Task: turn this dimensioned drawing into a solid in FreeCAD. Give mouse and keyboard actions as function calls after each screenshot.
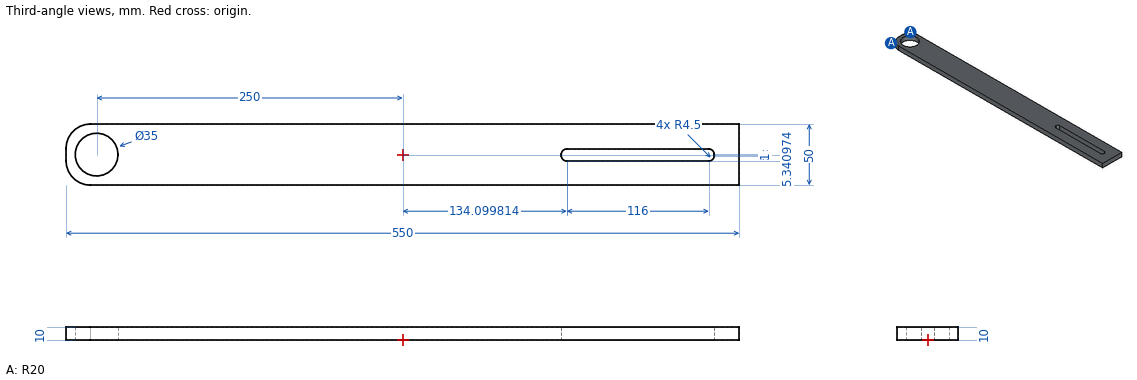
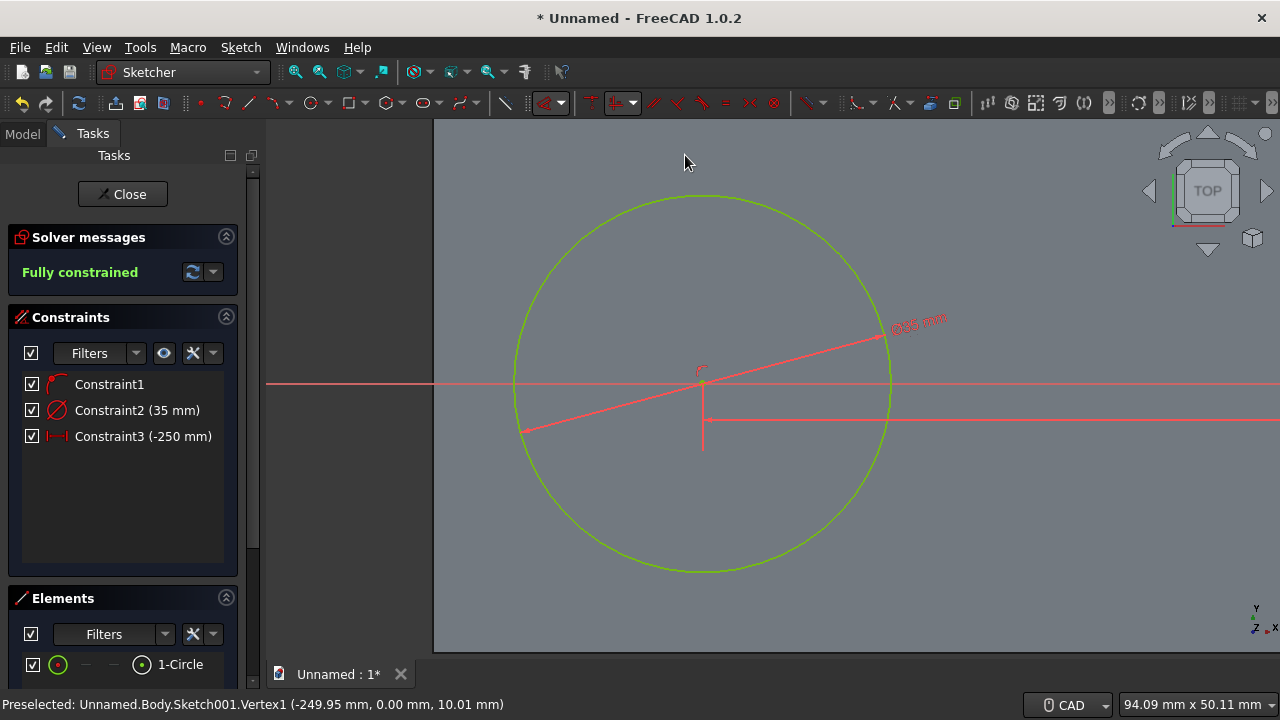
click(123, 194)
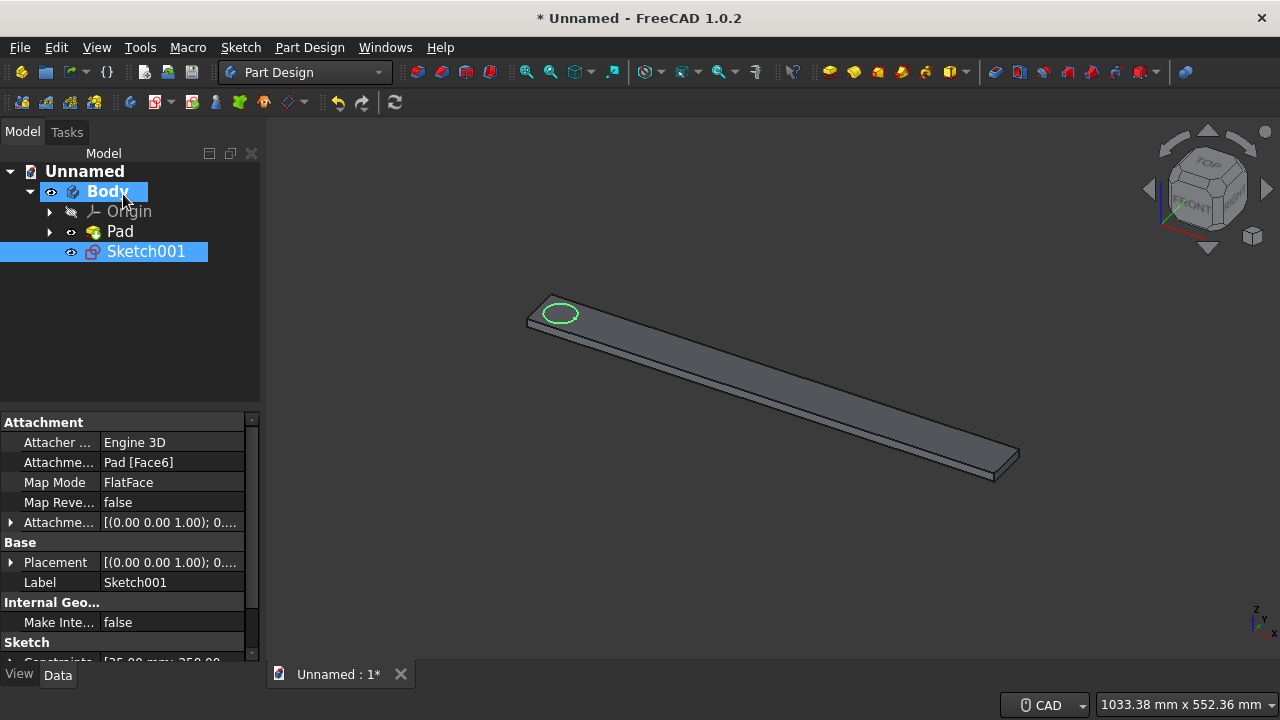
click(996, 72)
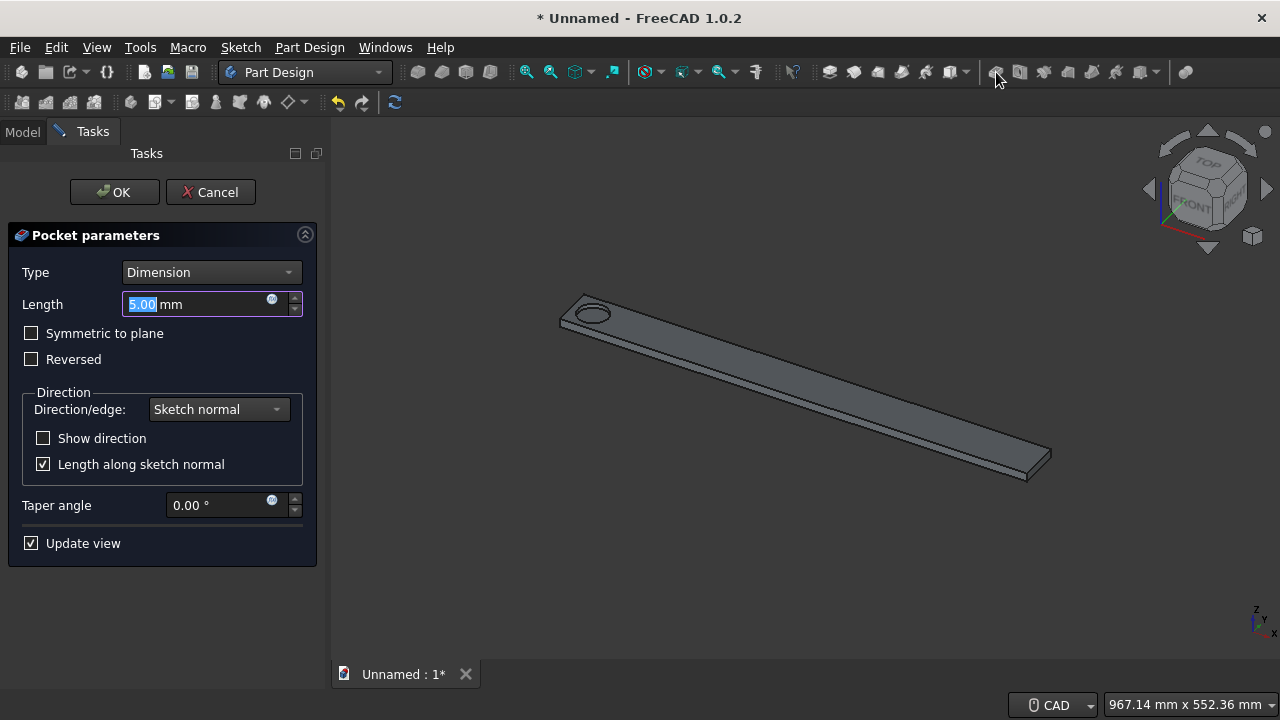
text(10)
key(Tab)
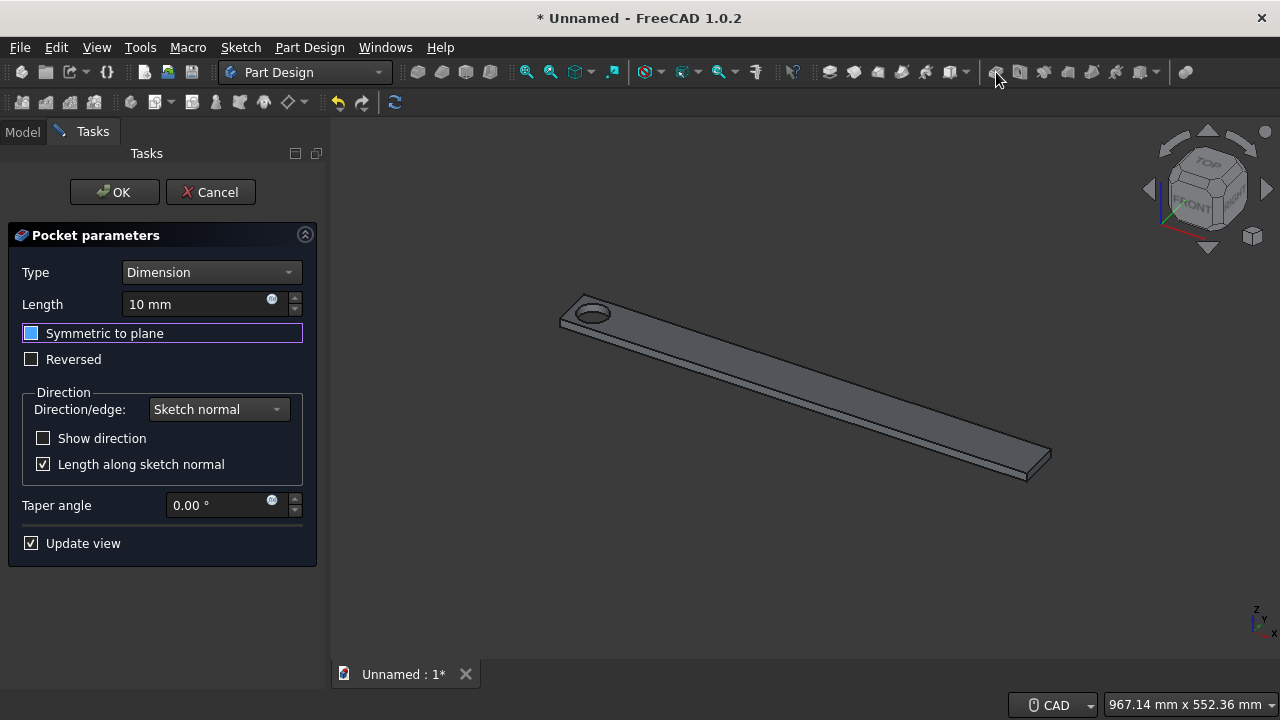
click(115, 192)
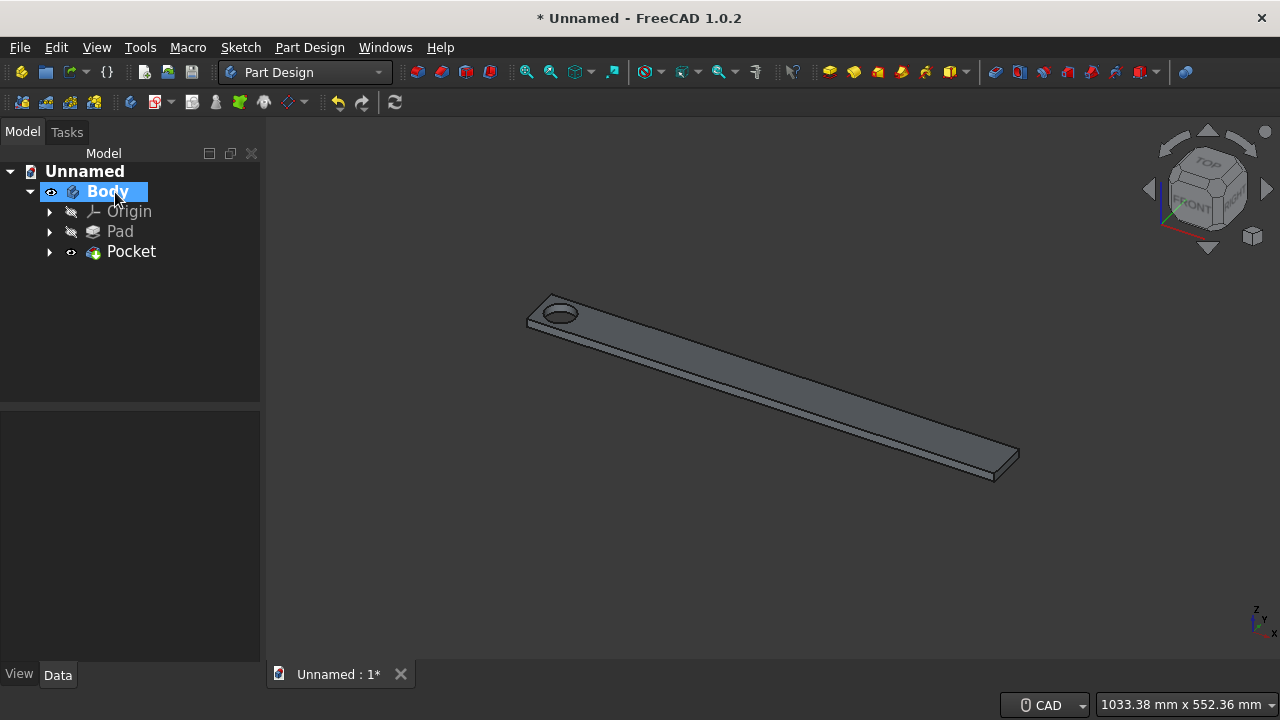
click(973, 449)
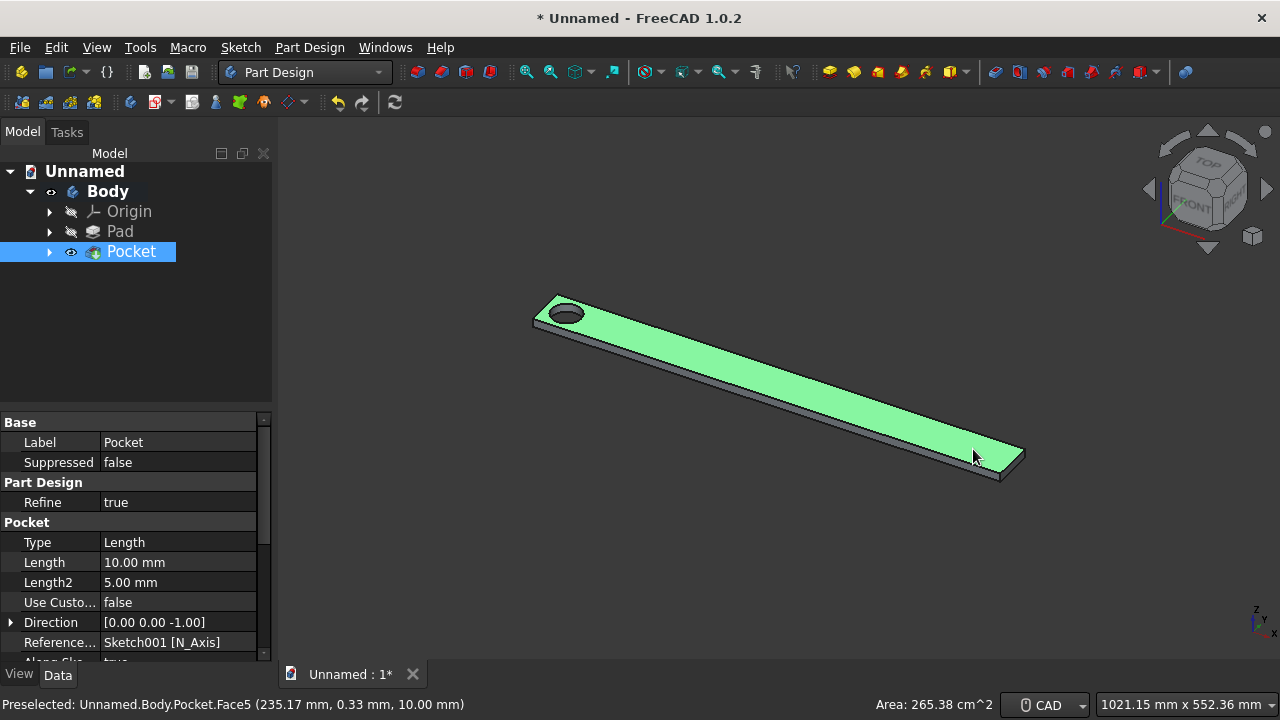
click(156, 102)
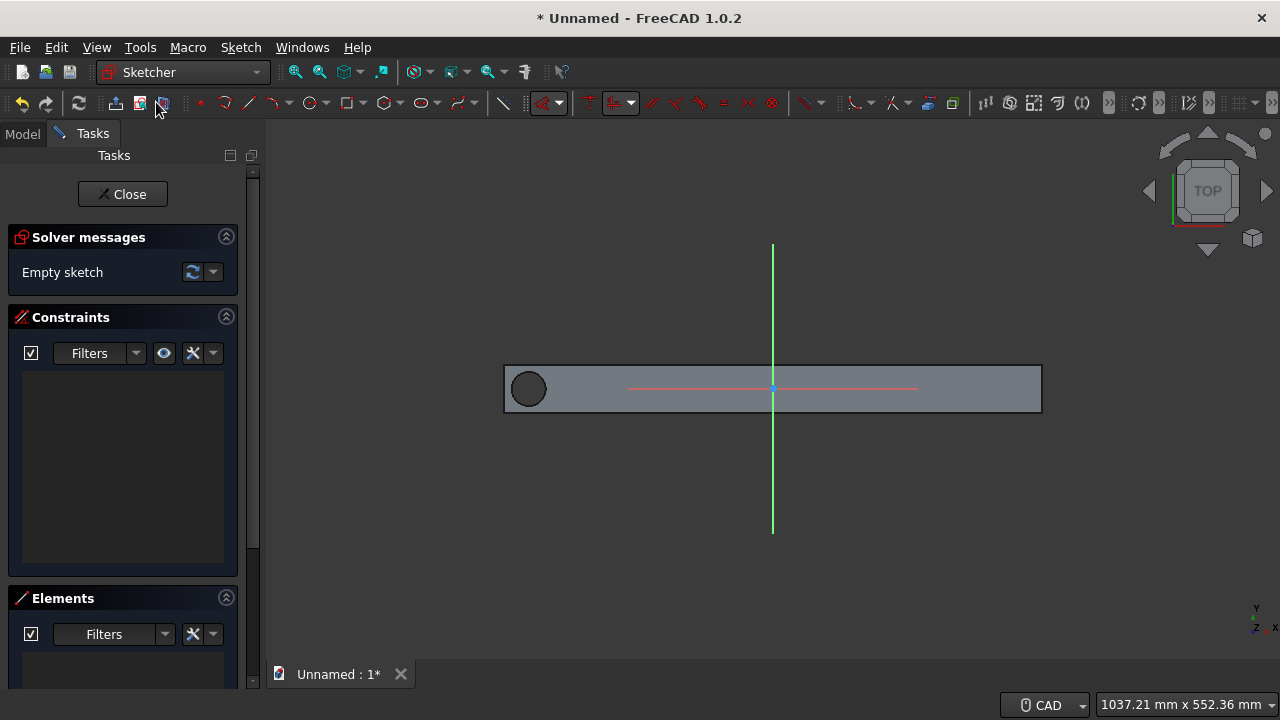
scroll(1055, 390, up, 4)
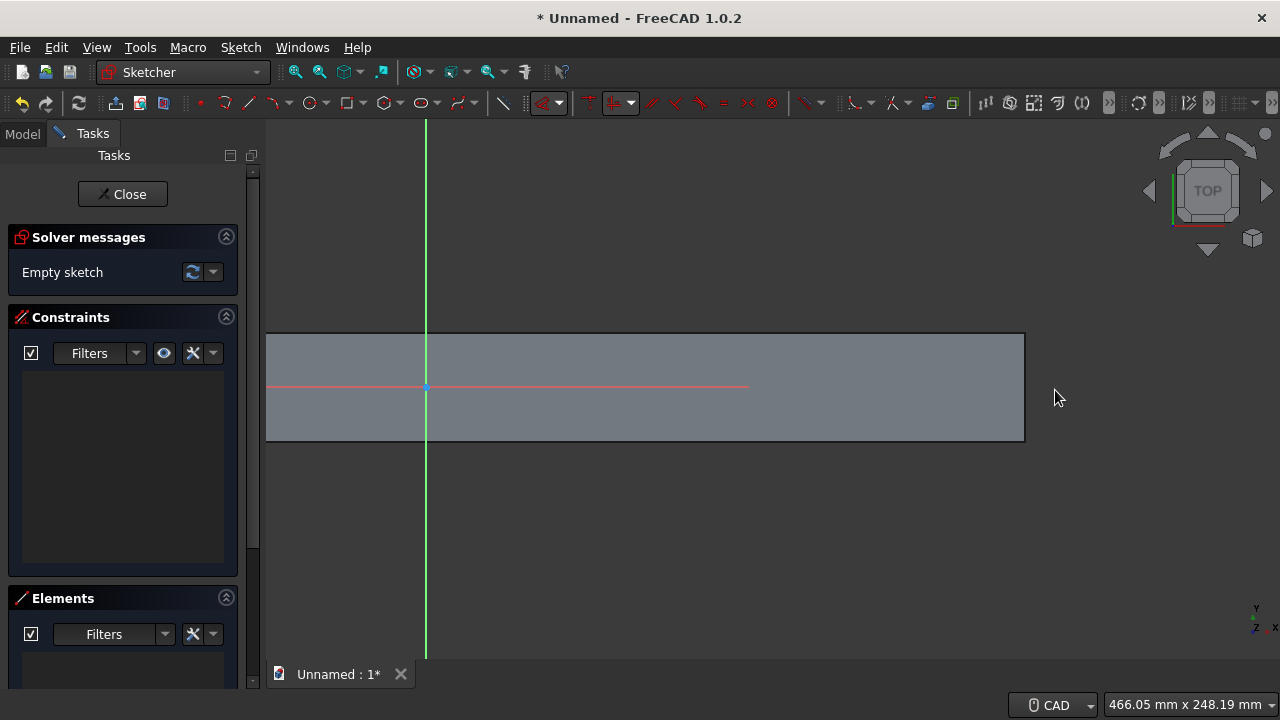
click(250, 104)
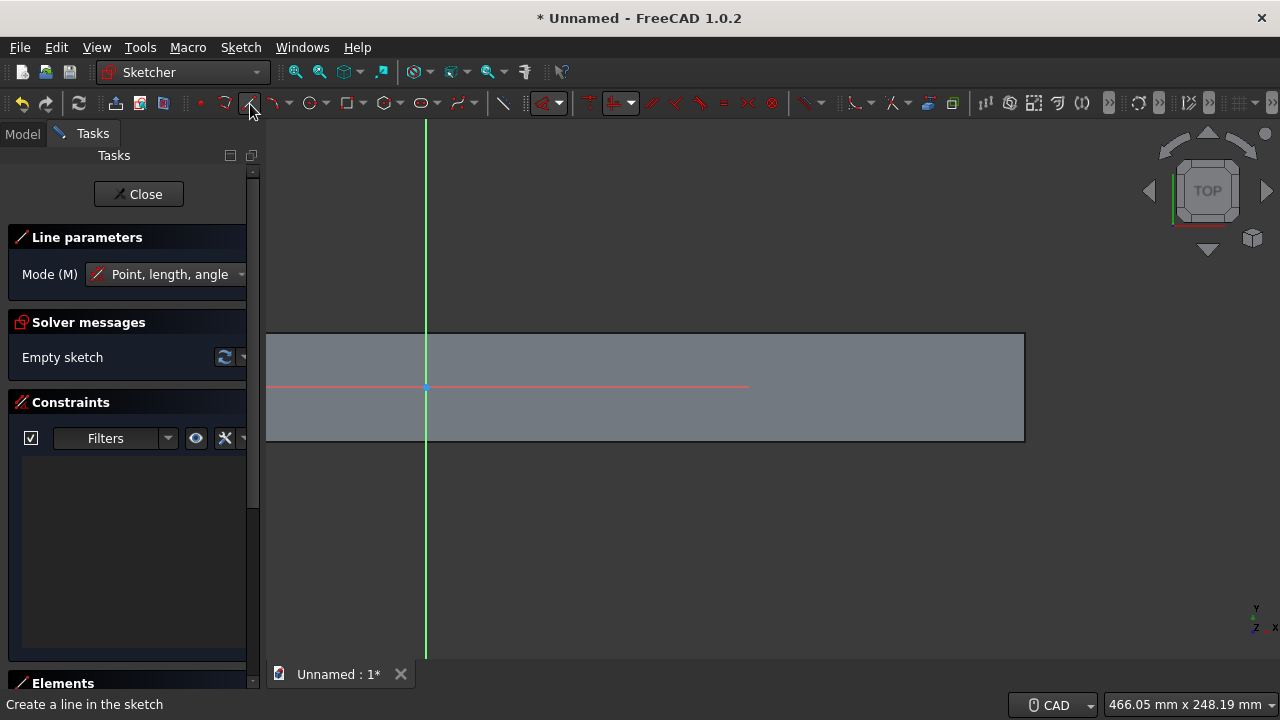
scroll(718, 399, up, 2)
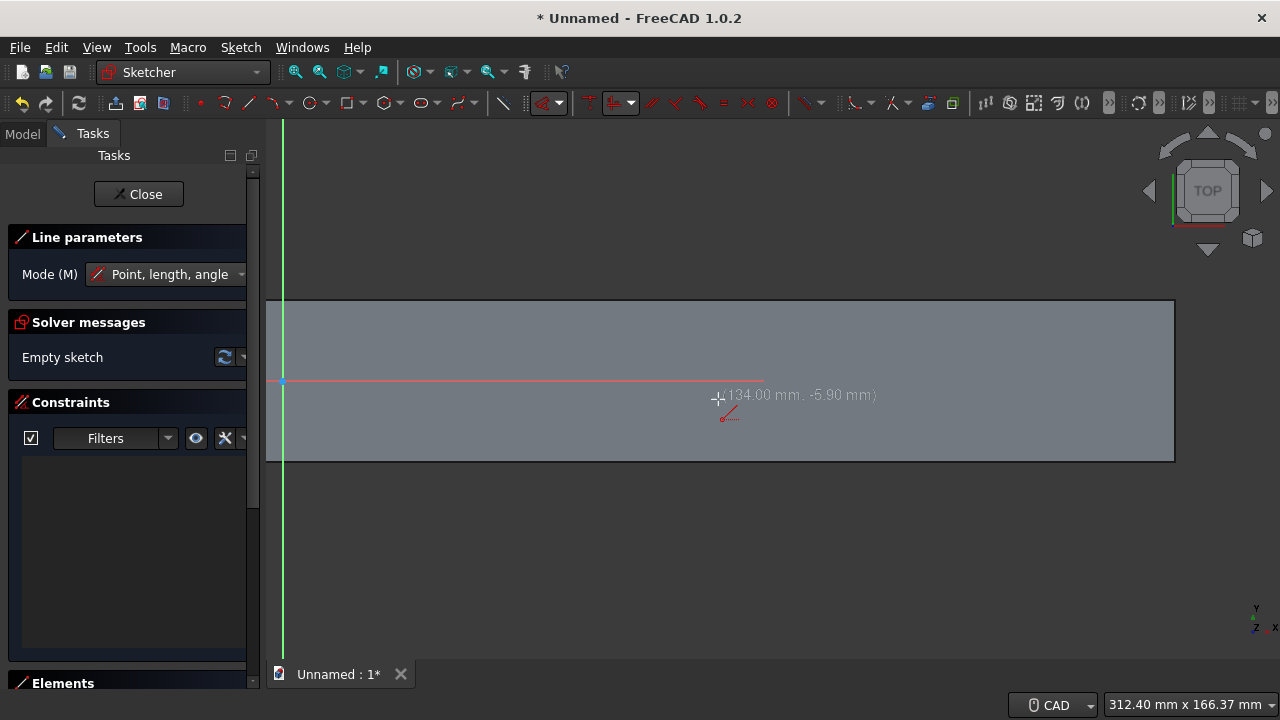
click(718, 398)
click(1095, 398)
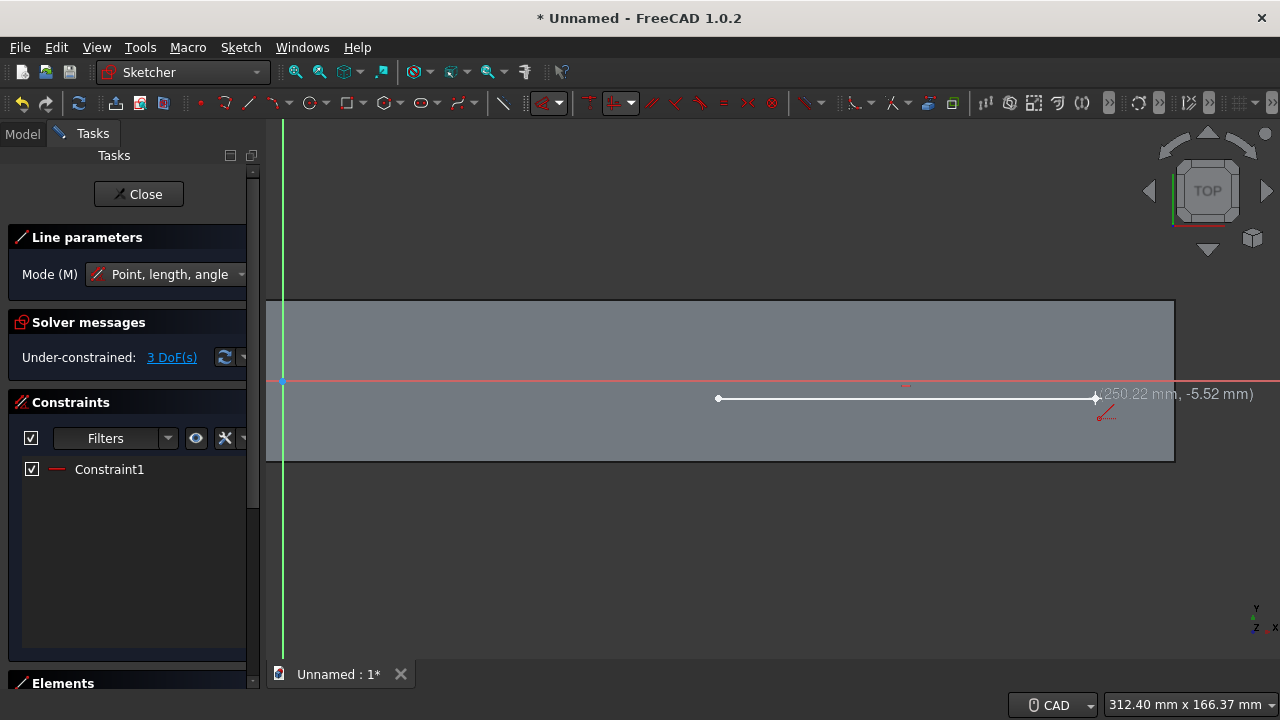
scroll(1109, 384, up, 9)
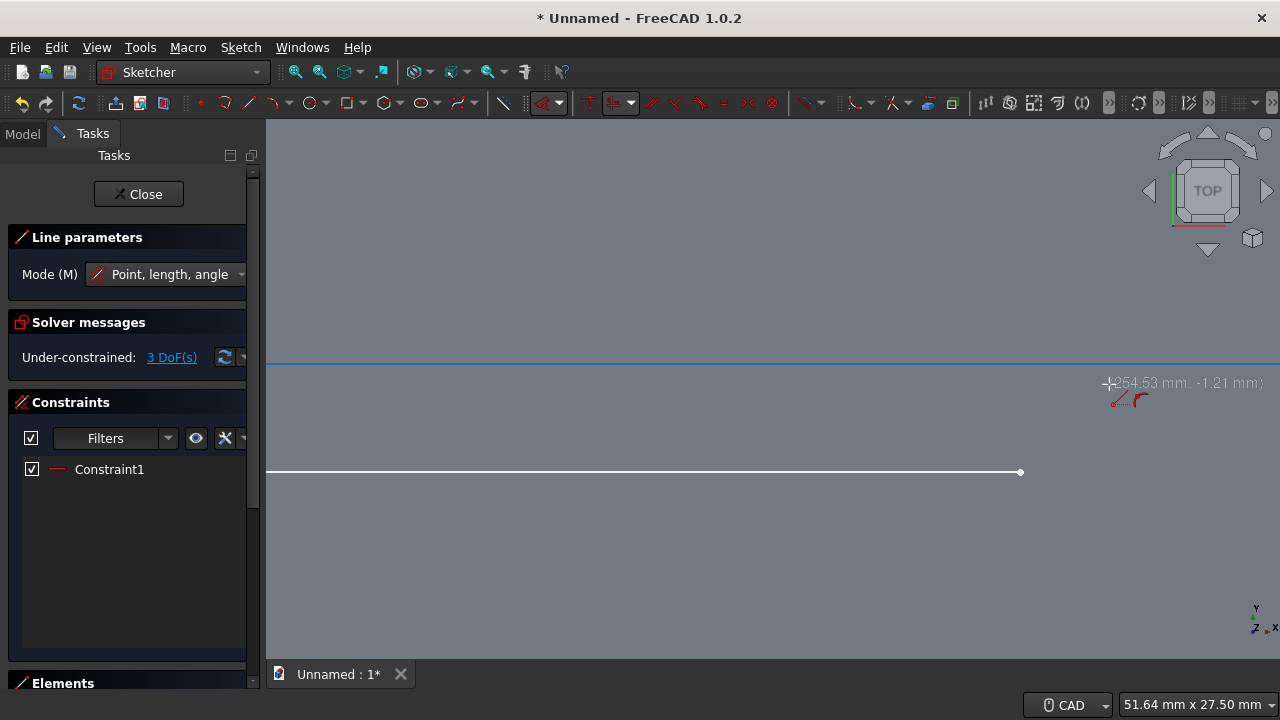
click(1106, 380)